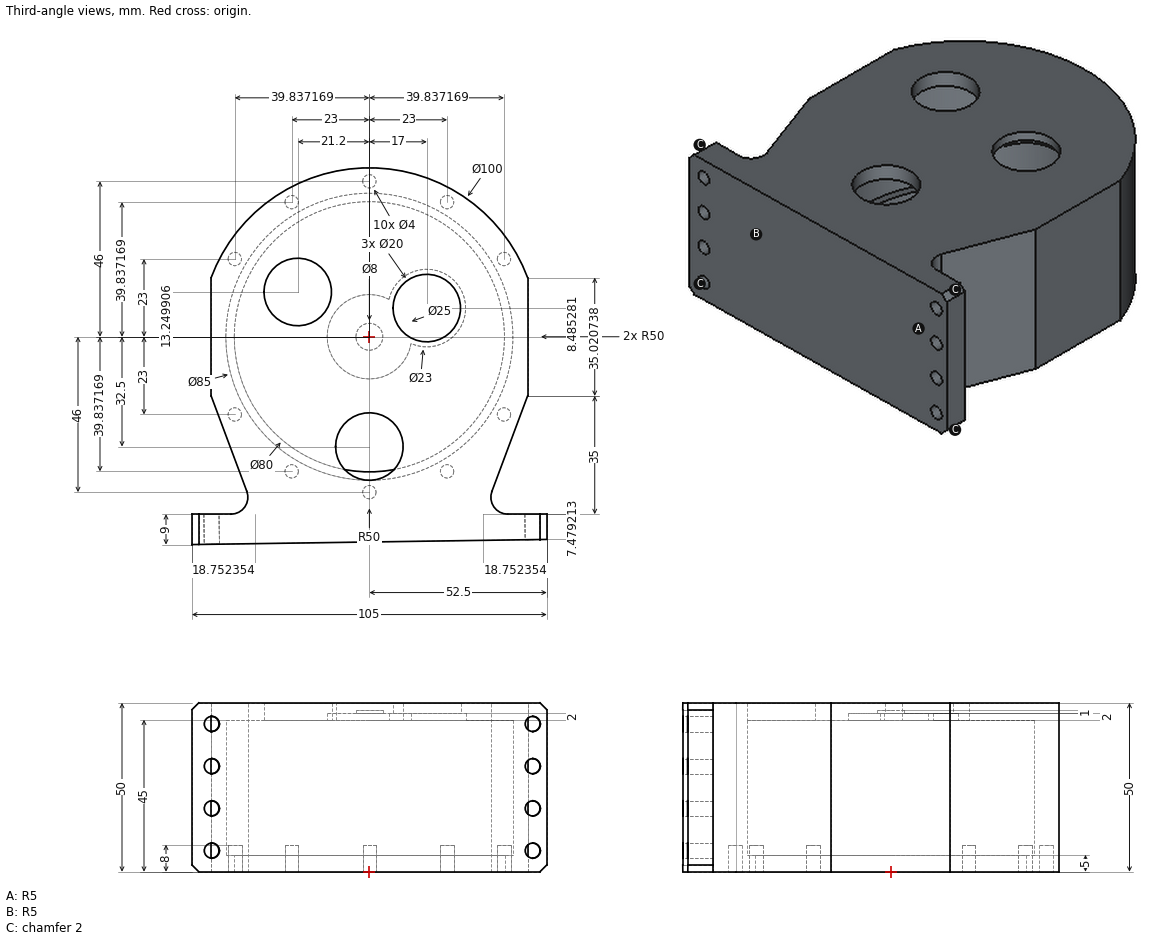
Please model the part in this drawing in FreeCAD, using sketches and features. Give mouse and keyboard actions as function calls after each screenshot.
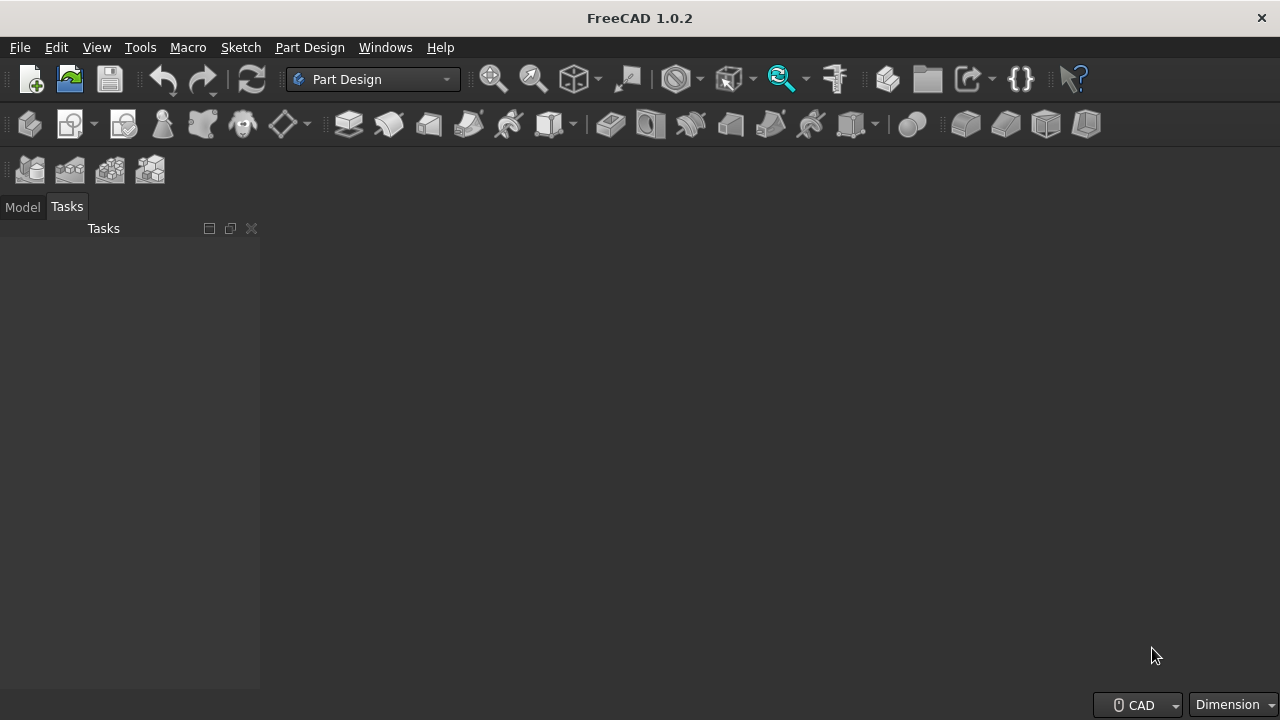
click(30, 80)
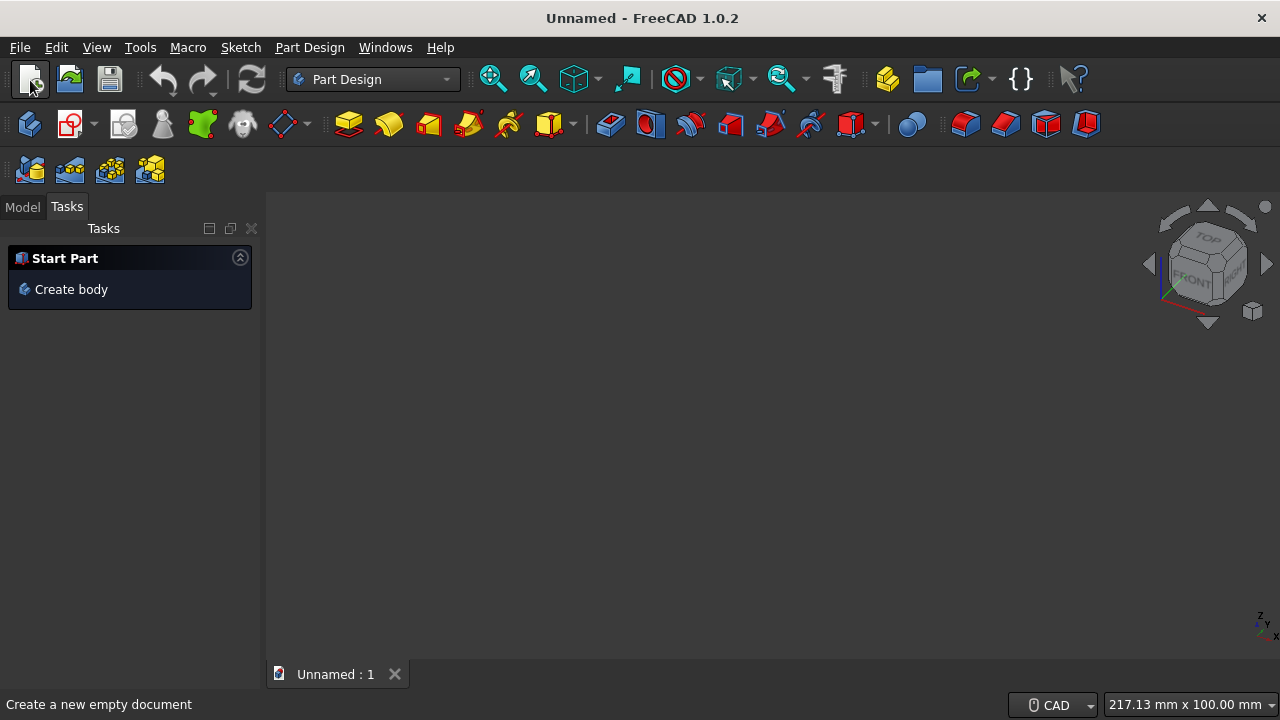
click(70, 124)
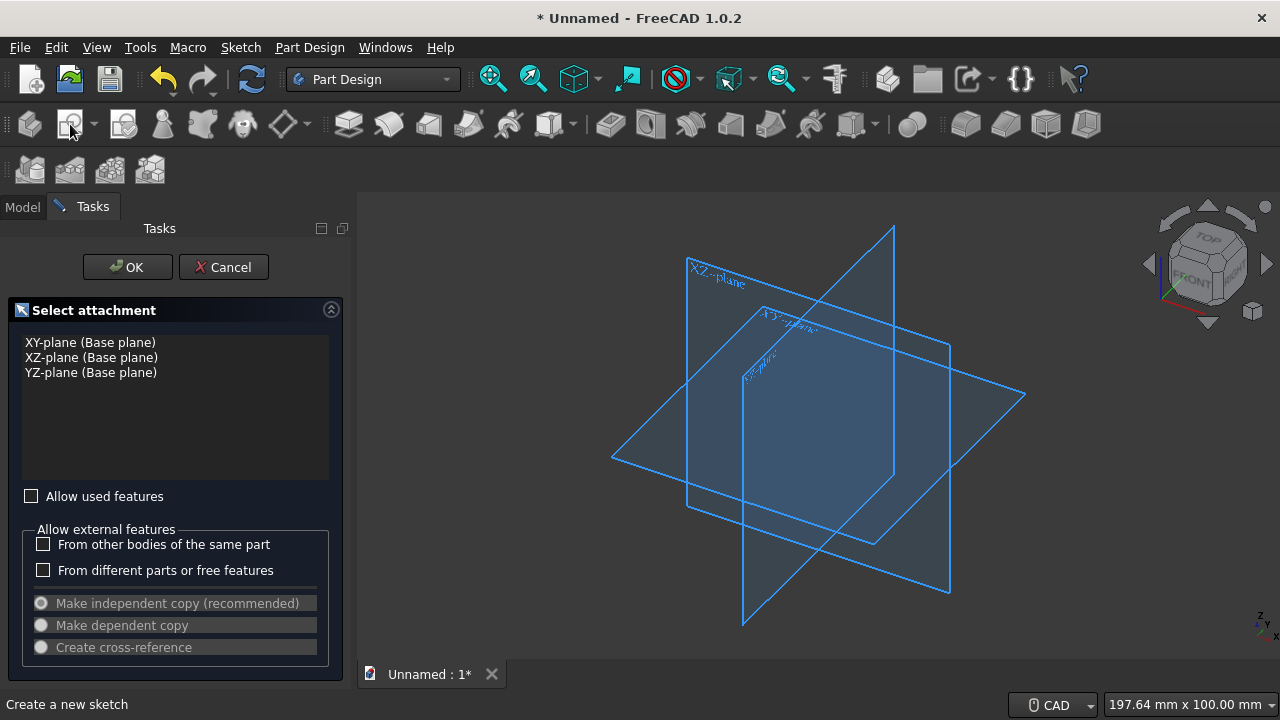
click(82, 342)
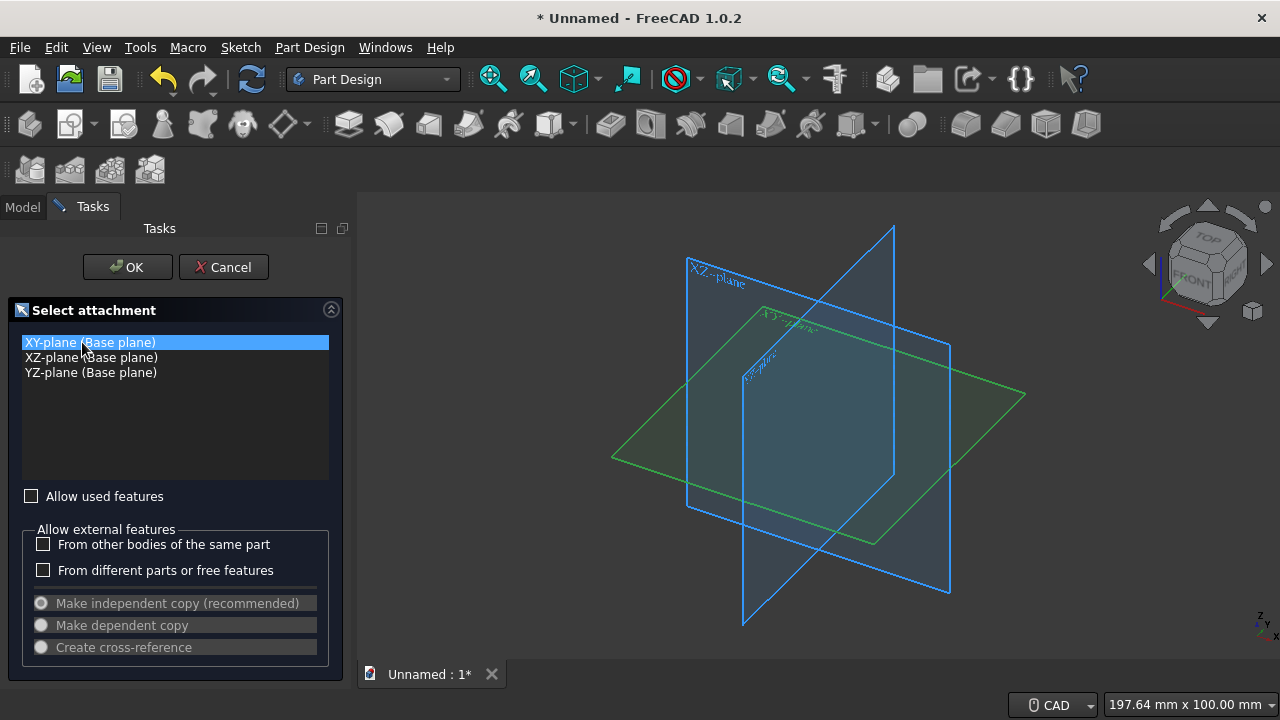
click(128, 267)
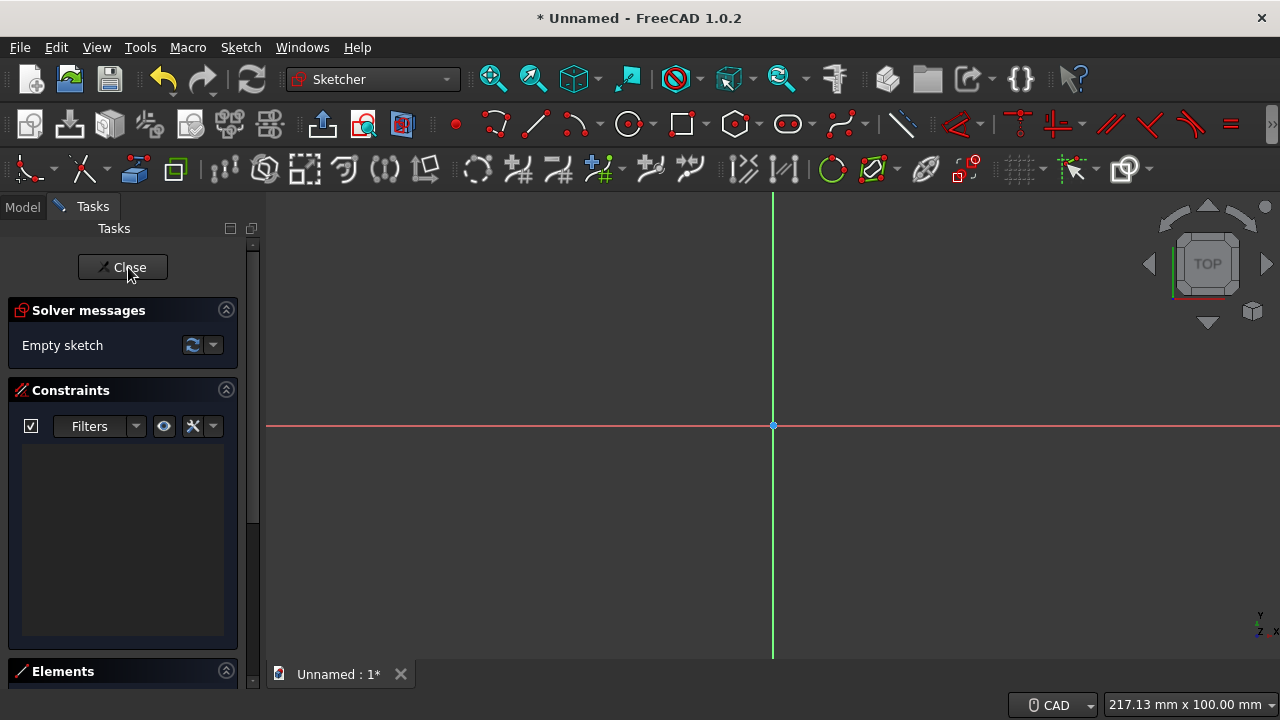
scroll(565, 425, down, 2)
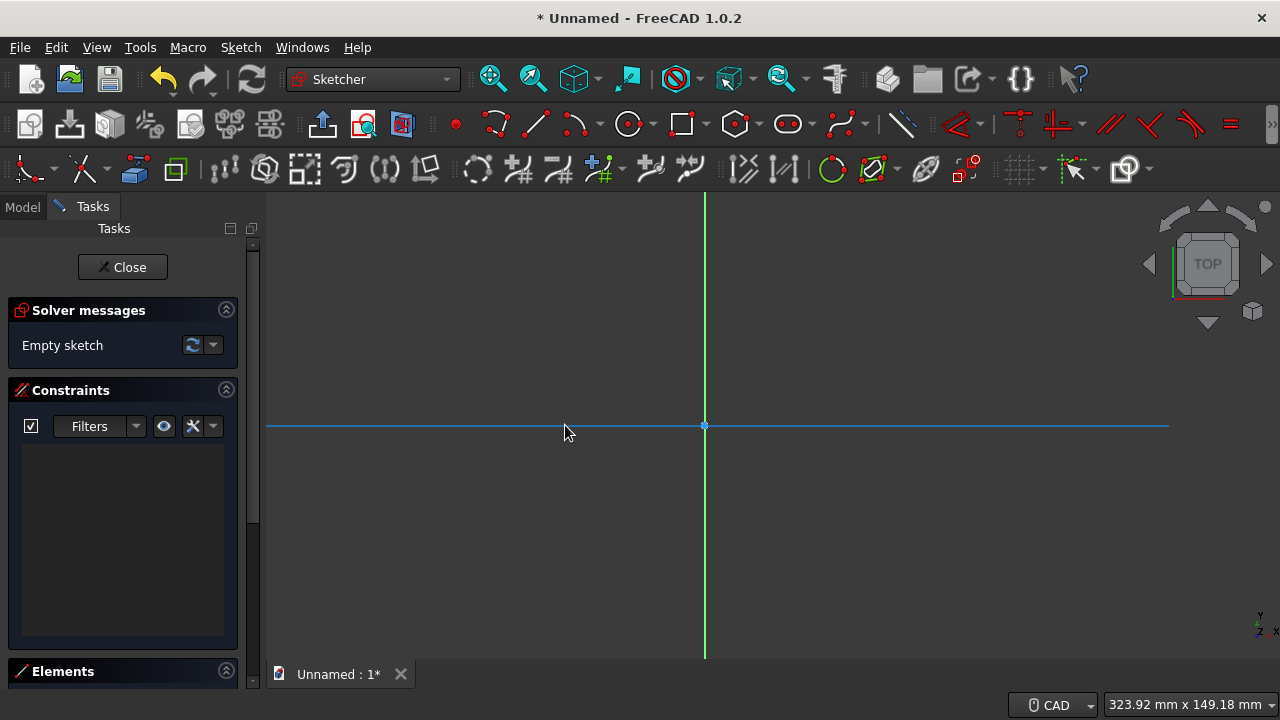
click(630, 124)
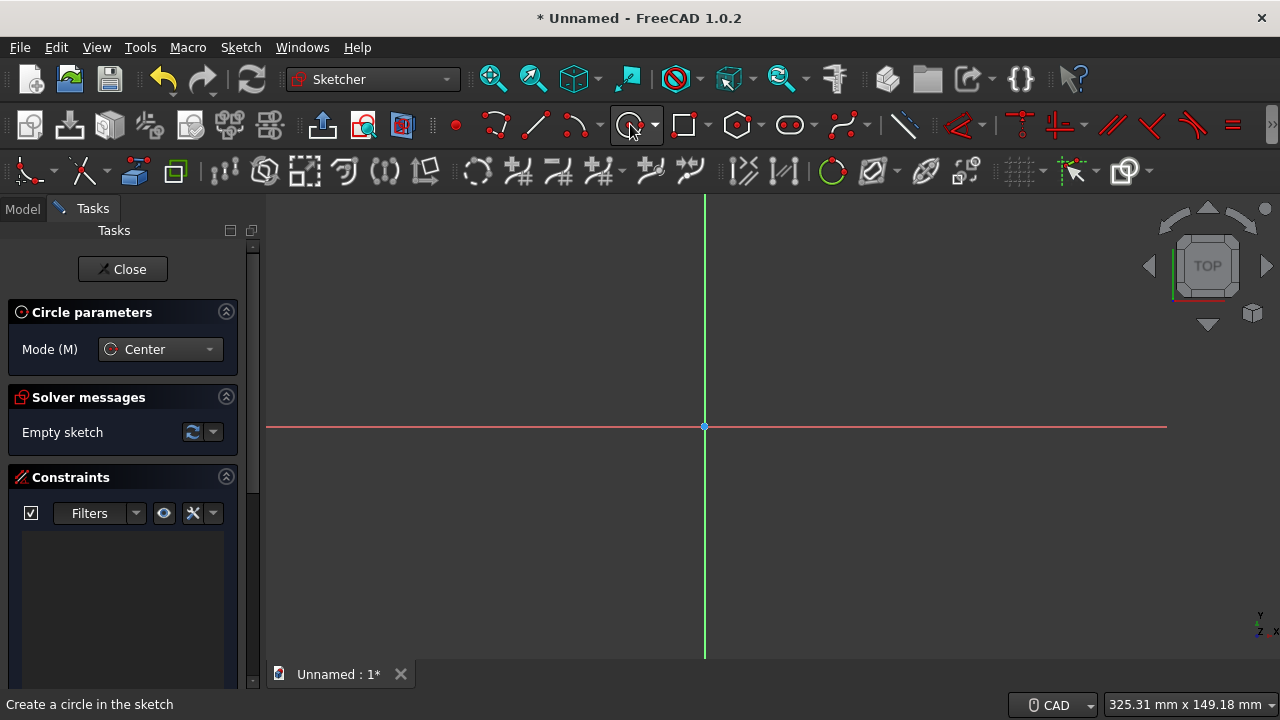
click(705, 426)
click(815, 316)
key(Escape)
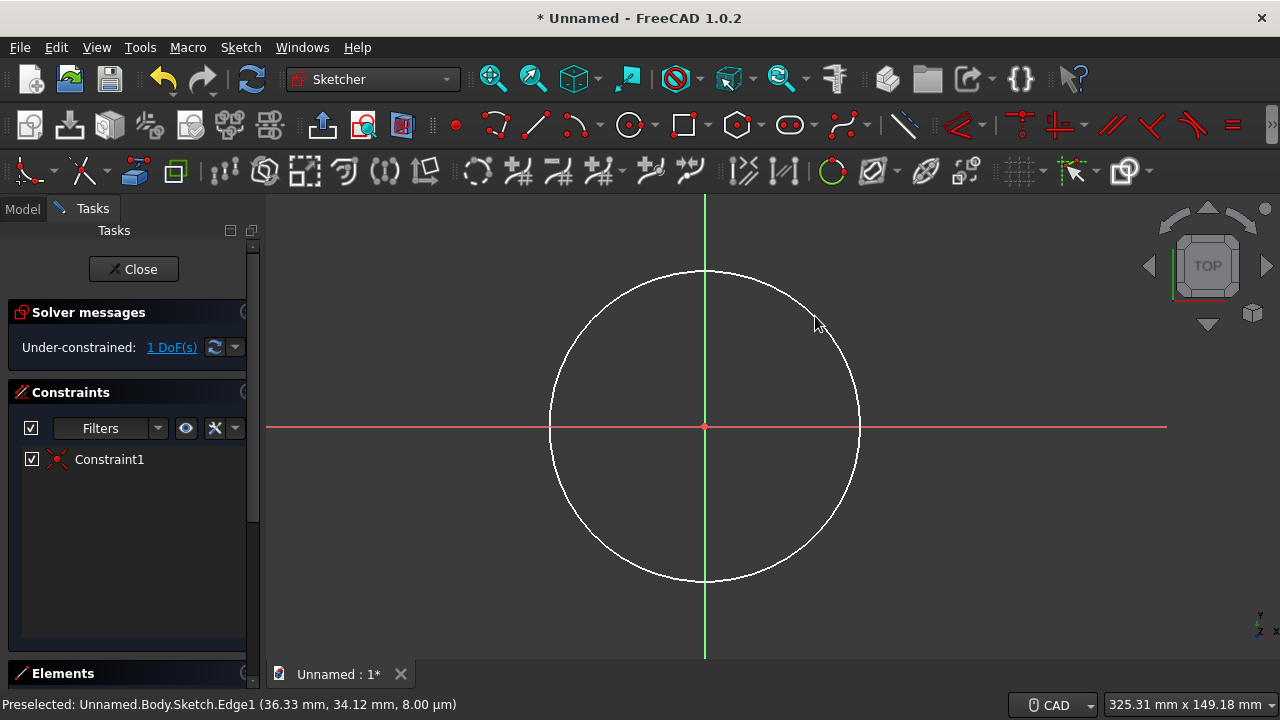
click(958, 126)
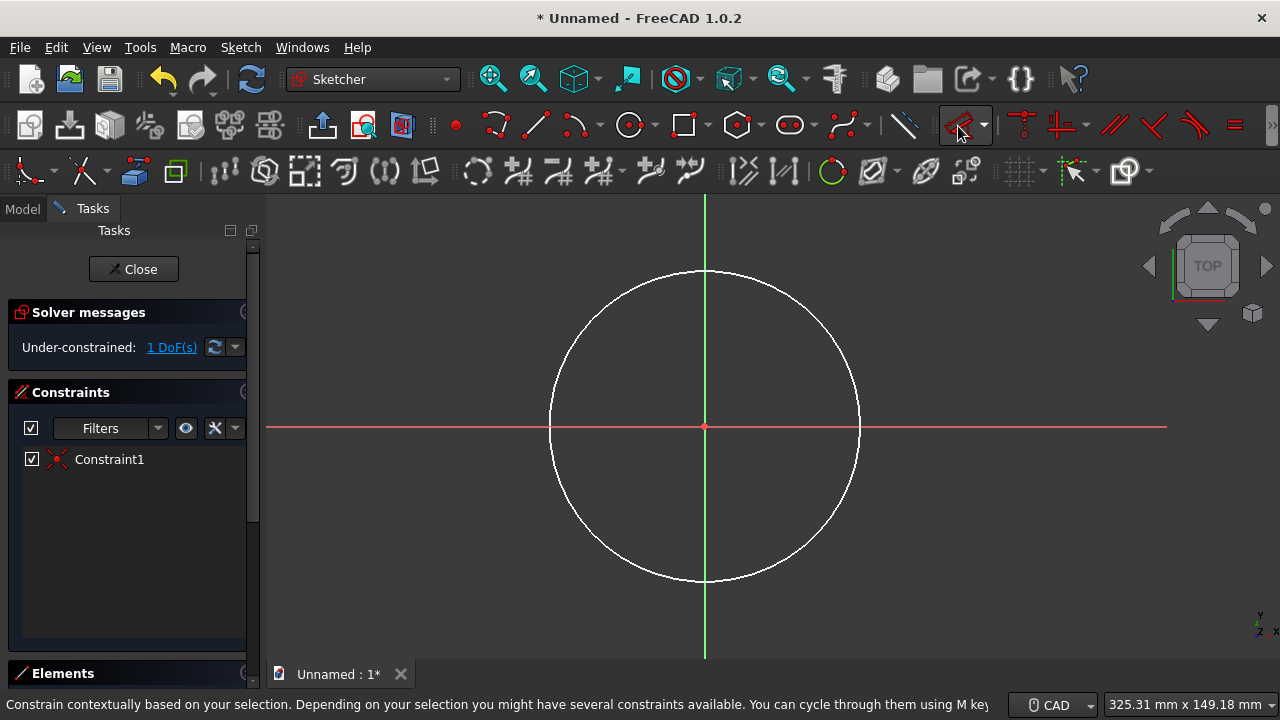
click(814, 316)
click(836, 293)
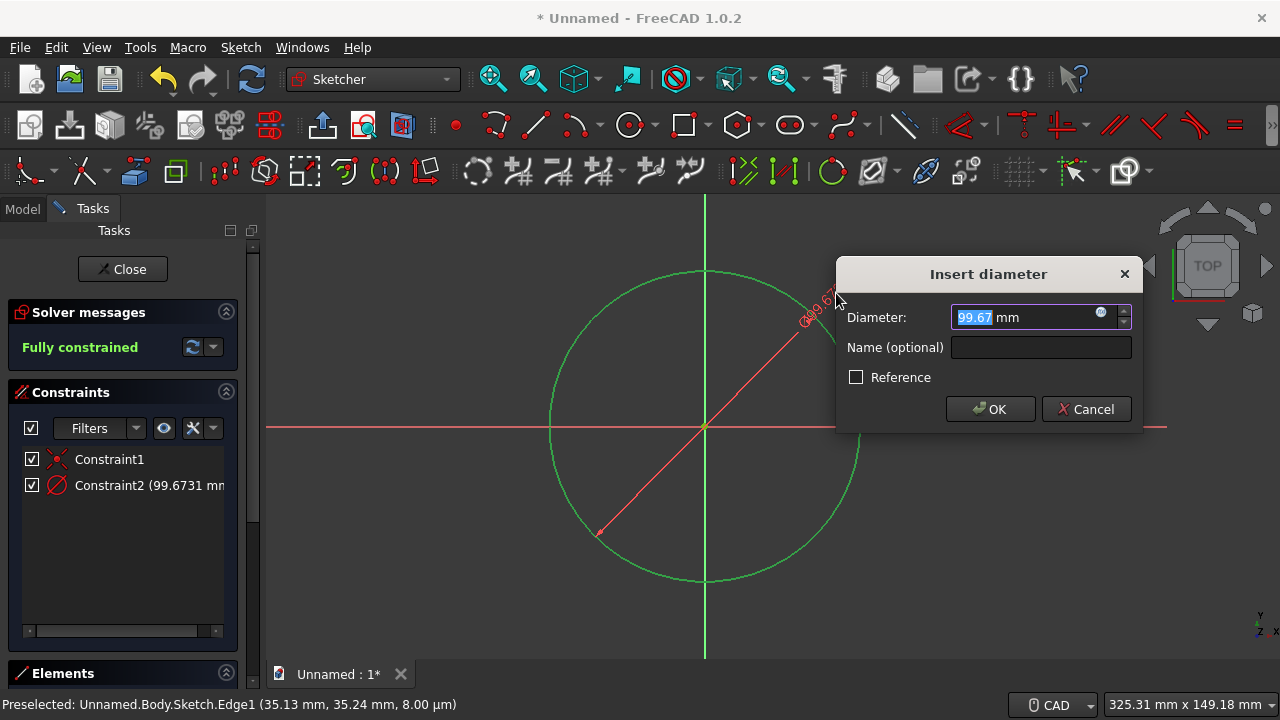
text(100)
key(Return)
key(Escape)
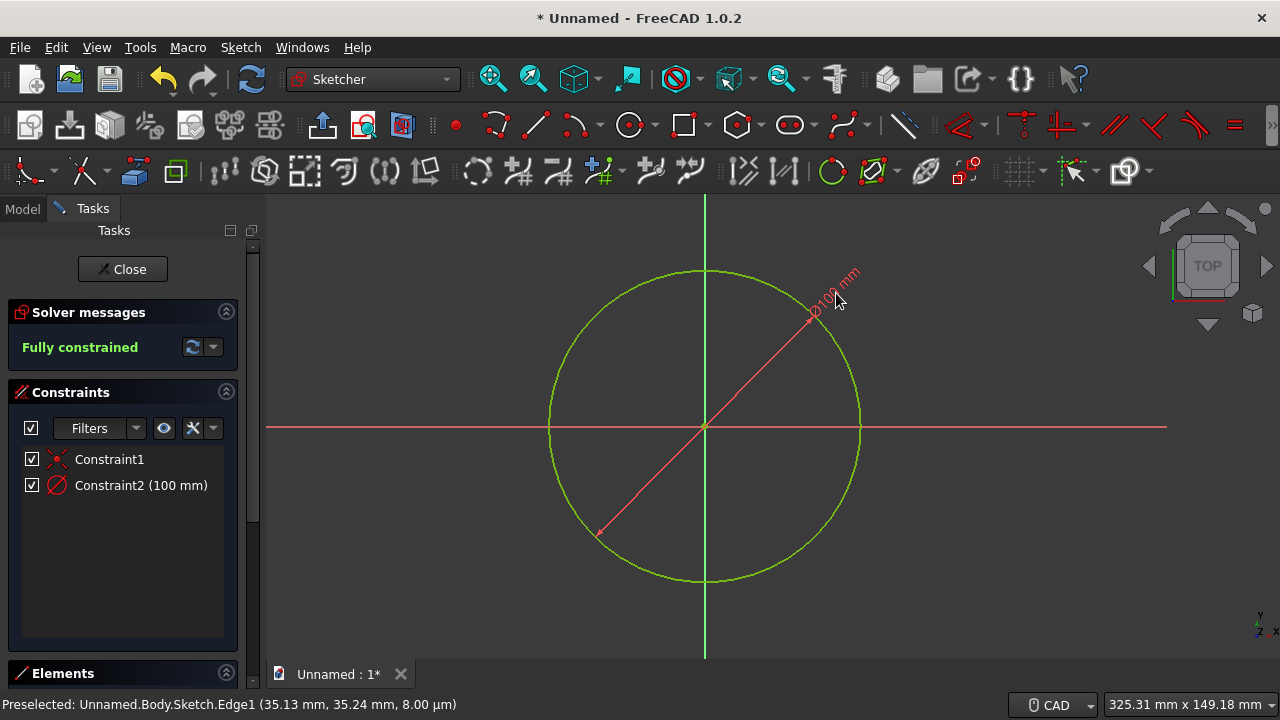
click(123, 269)